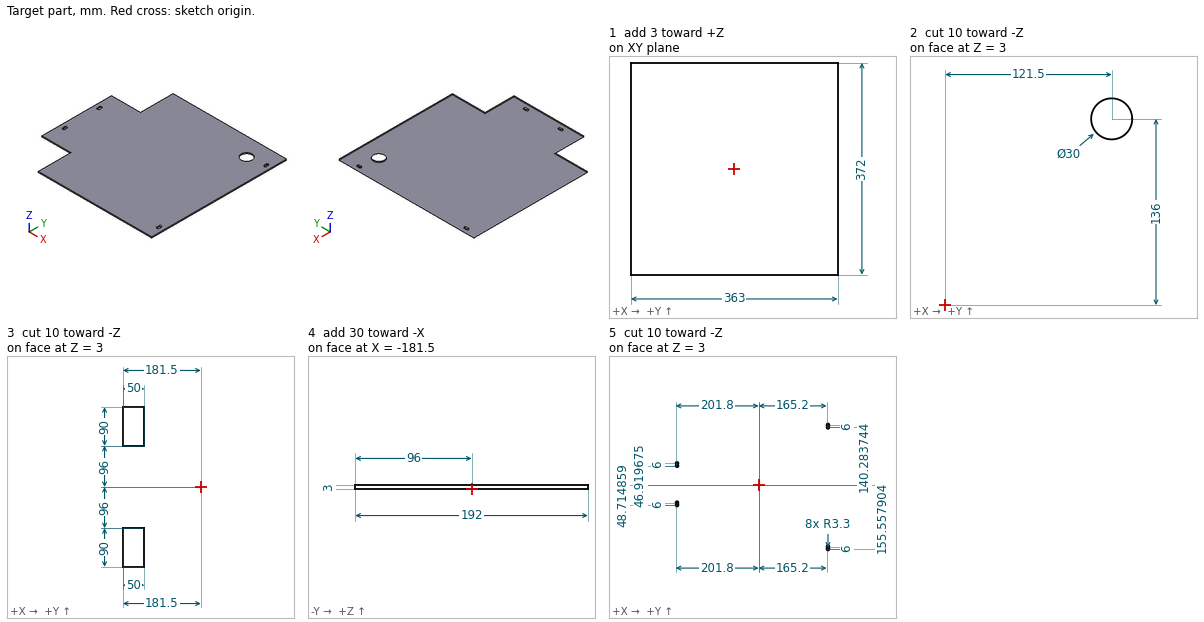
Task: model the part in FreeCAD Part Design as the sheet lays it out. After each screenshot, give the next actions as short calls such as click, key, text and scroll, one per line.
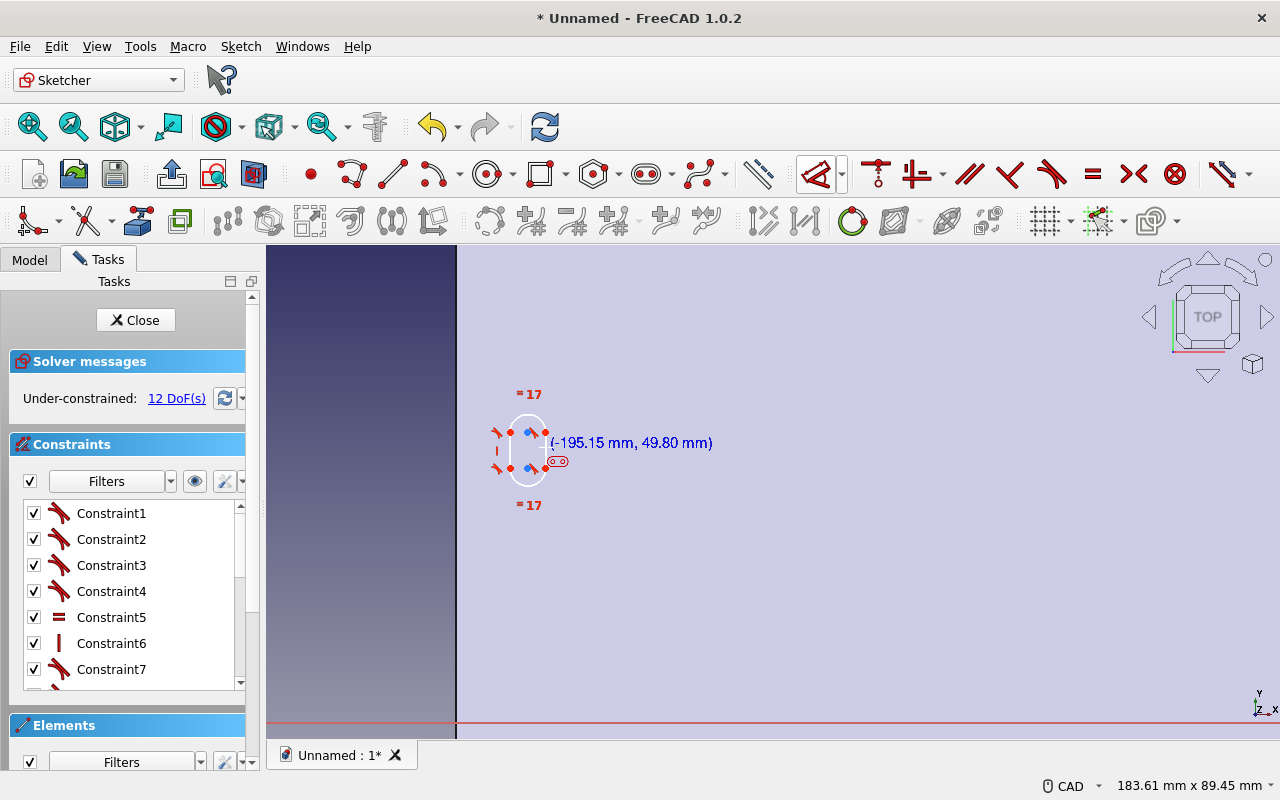
scroll(539, 441, down, 9)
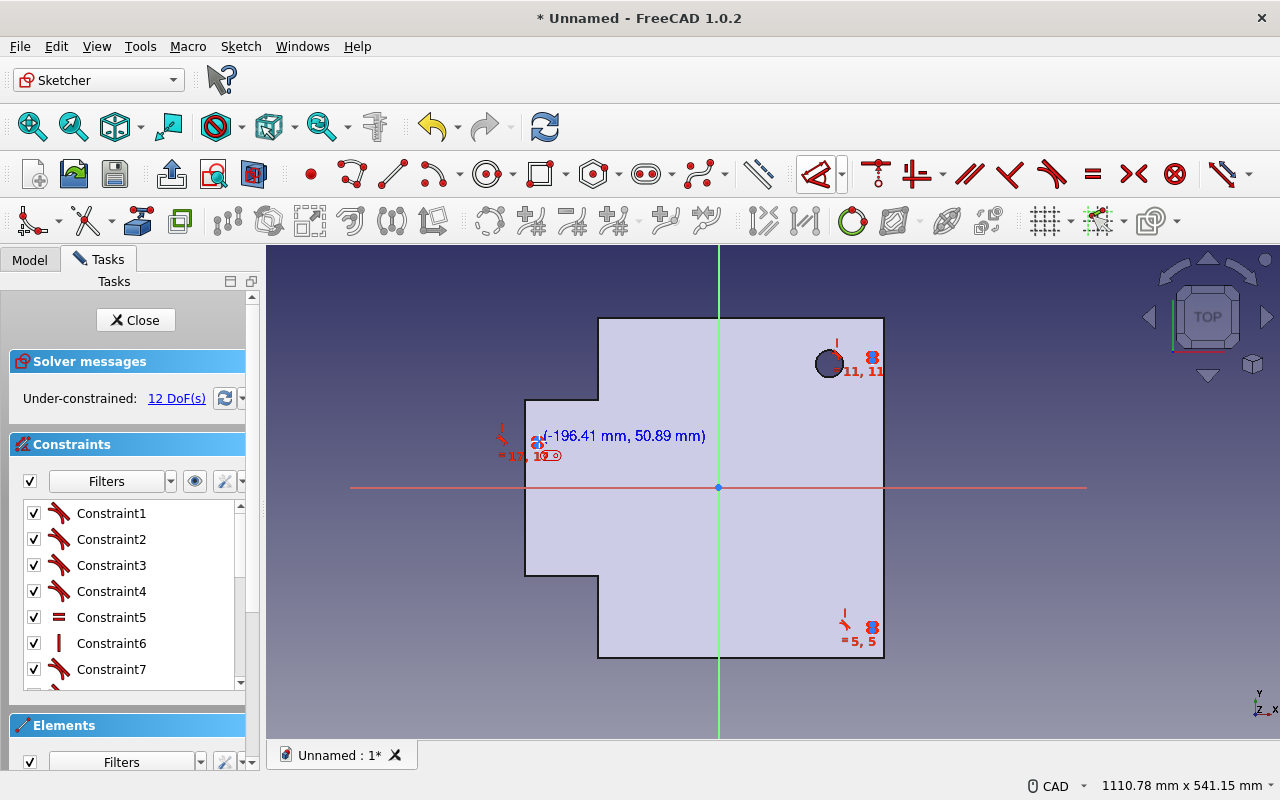
scroll(537, 532, up, 11)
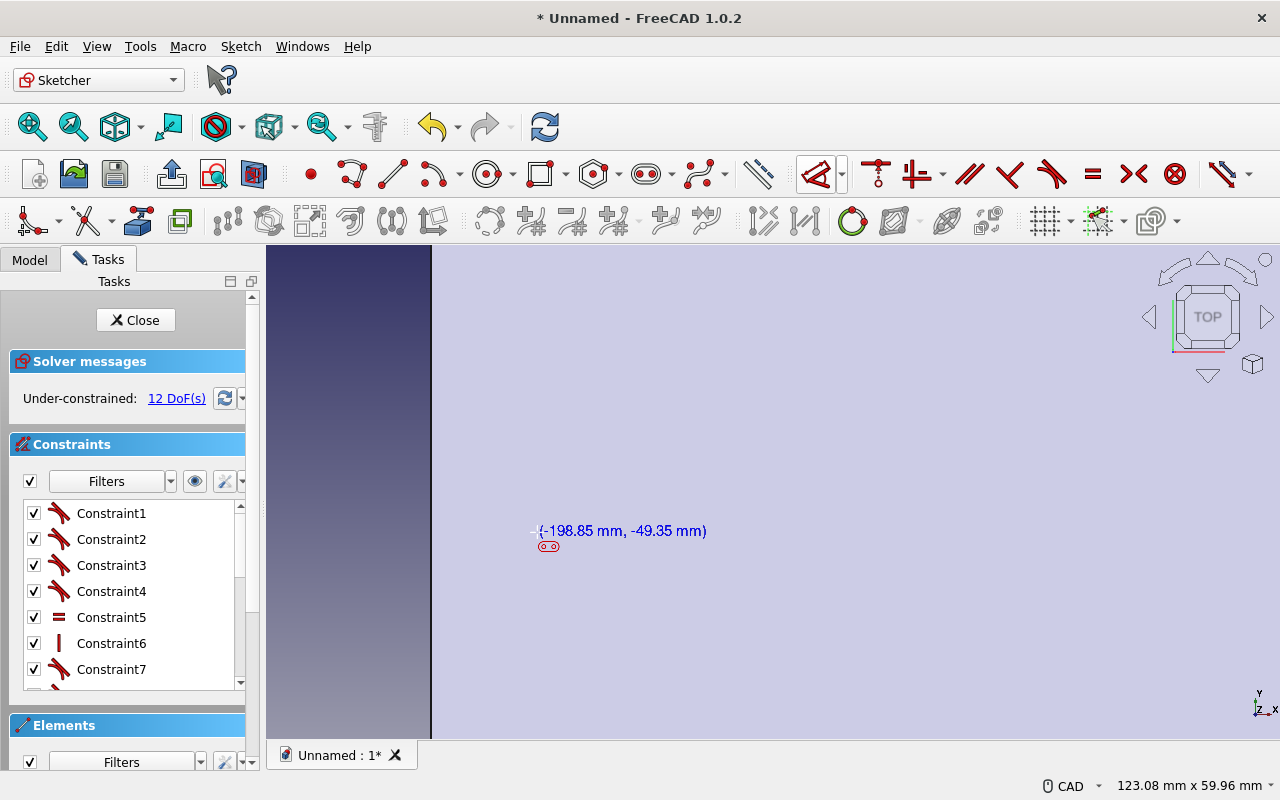
scroll(537, 532, down, 11)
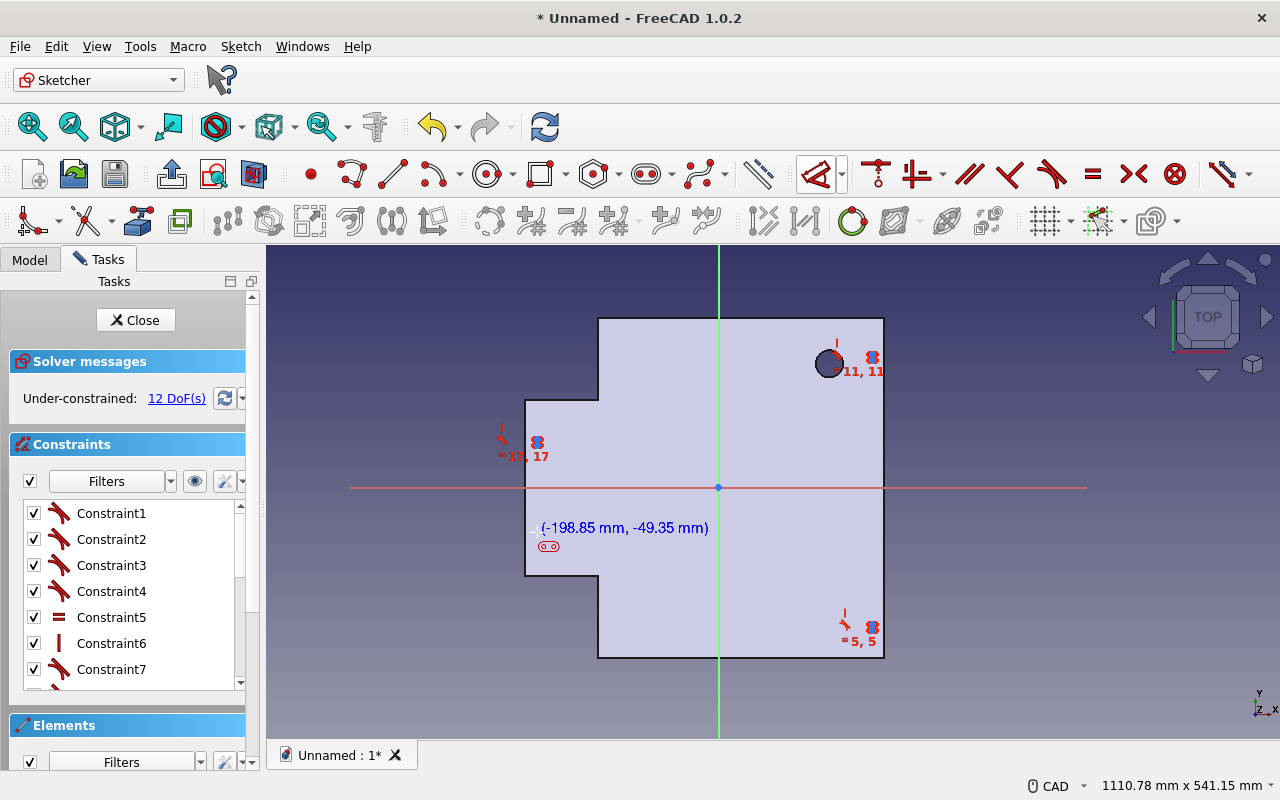
click(537, 532)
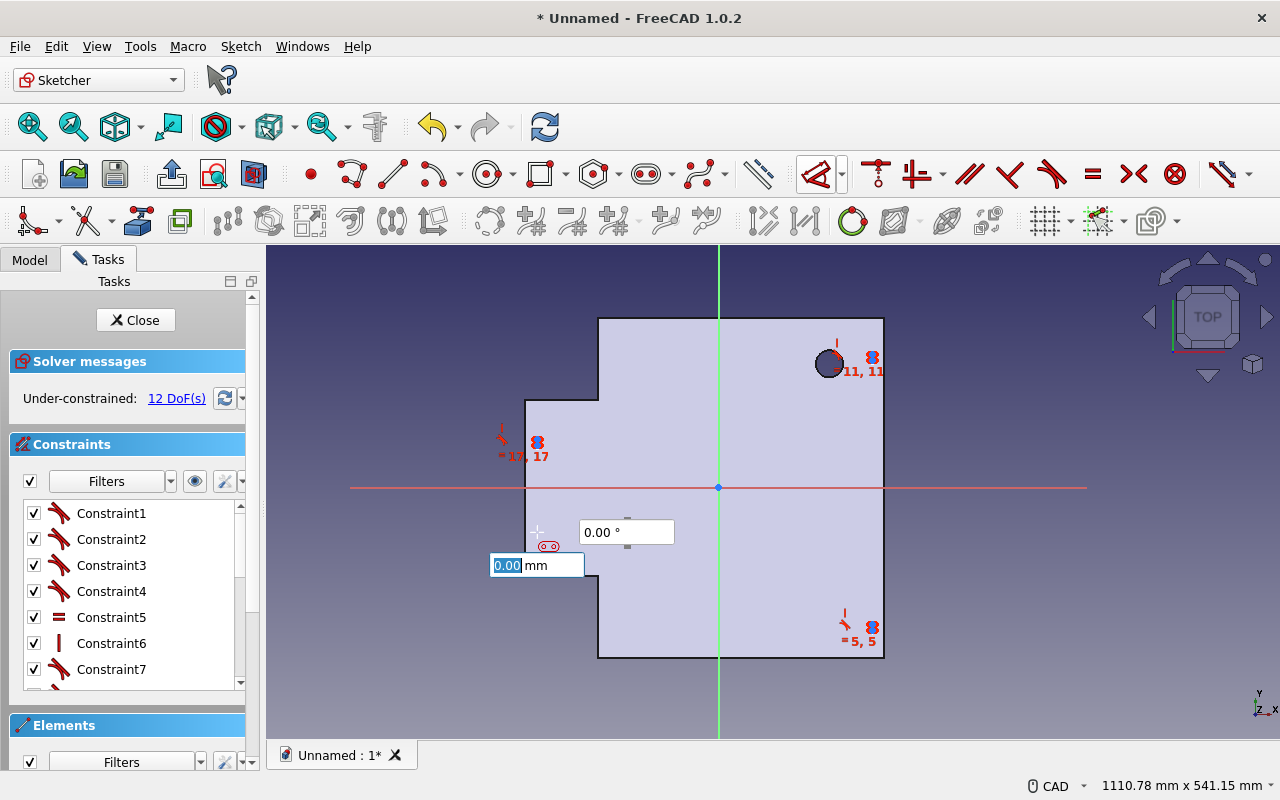
scroll(537, 527, up, 6)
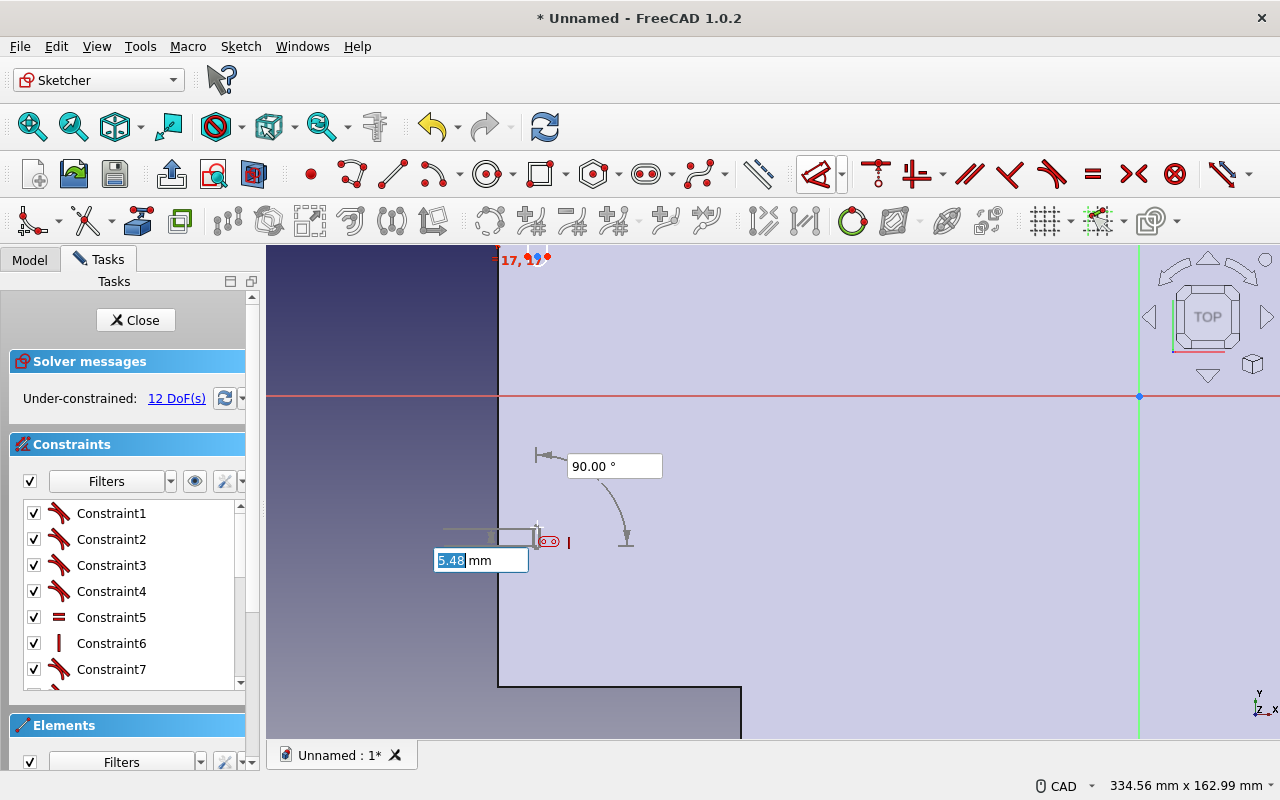
click(536, 525)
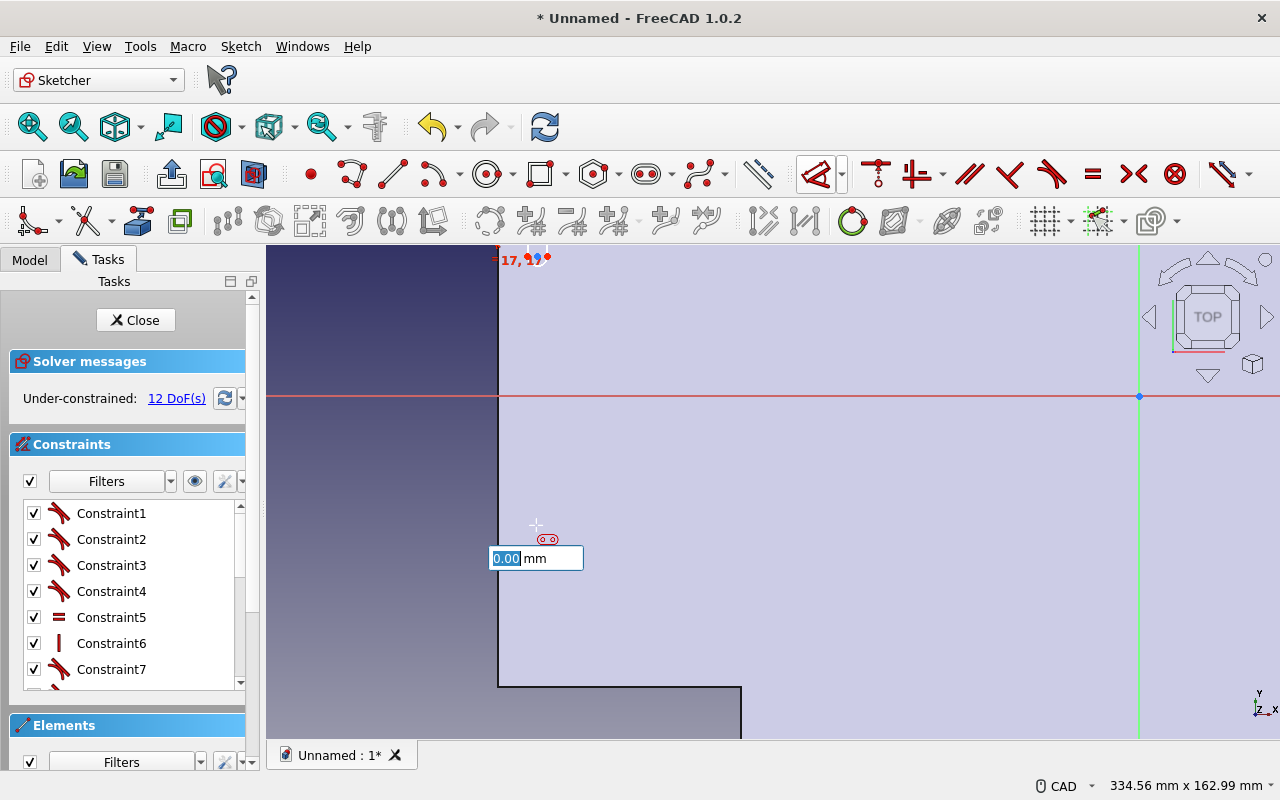
scroll(527, 535, up, 3)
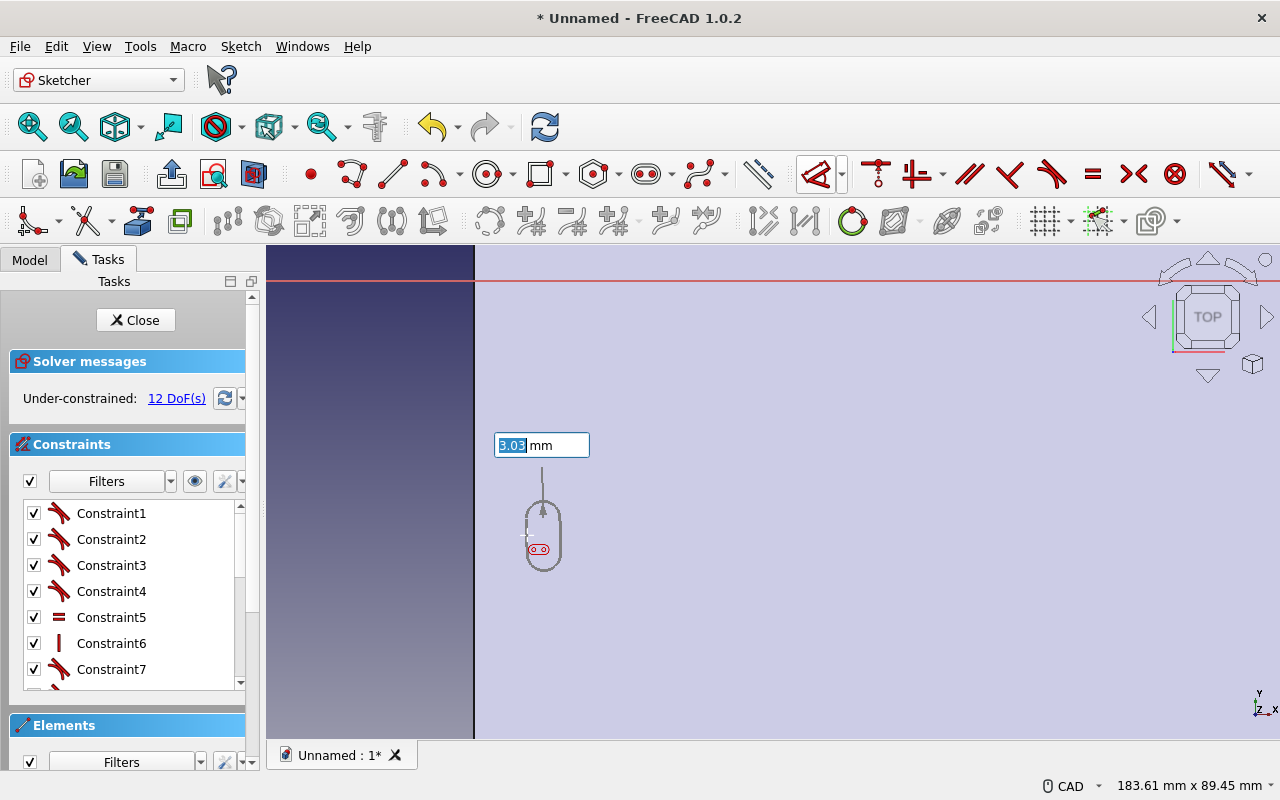
click(528, 534)
key(Escape)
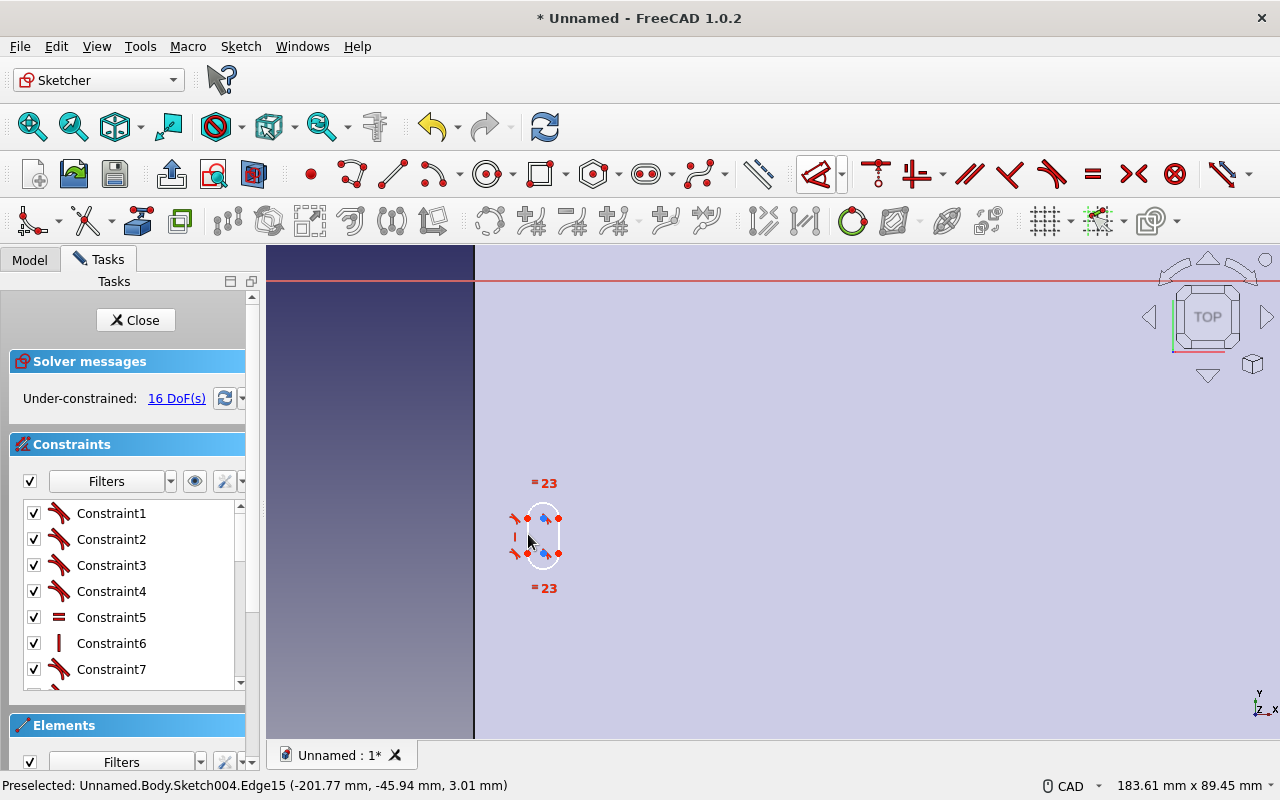
scroll(535, 529, down, 9)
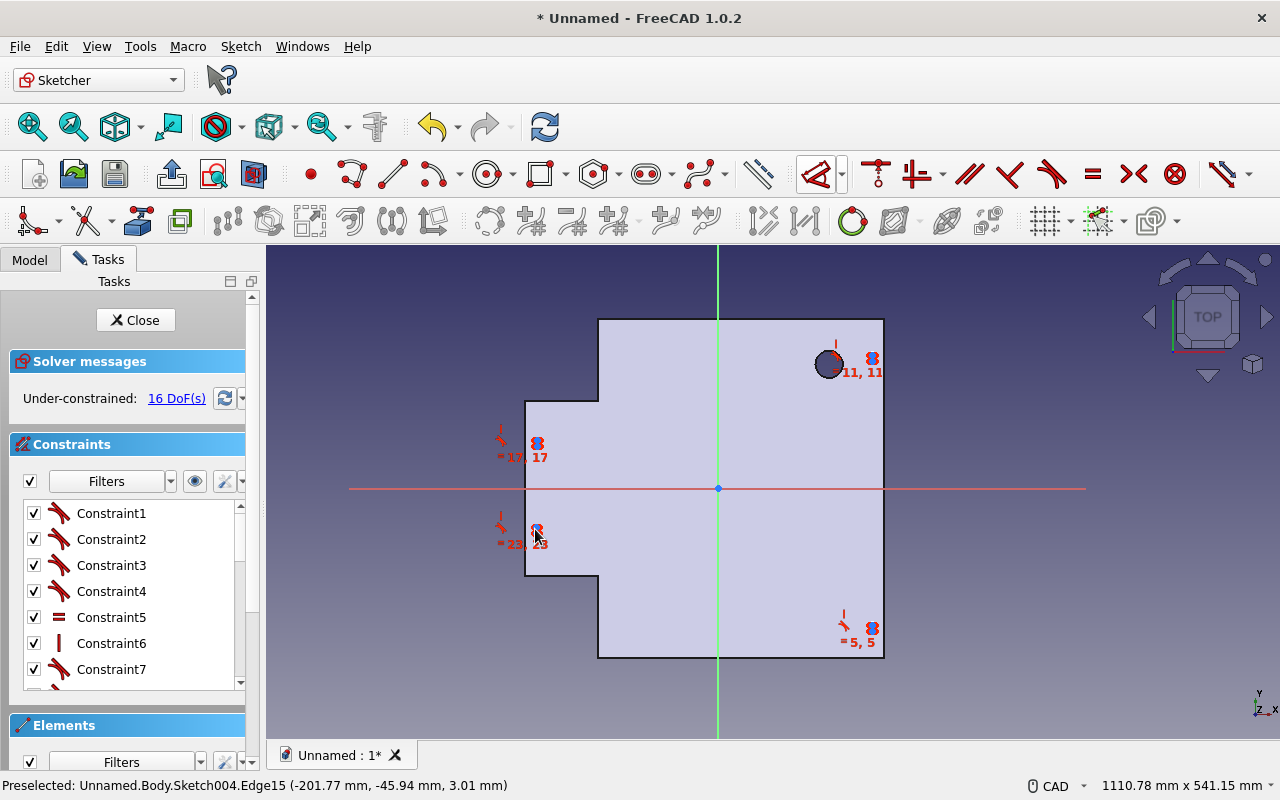
scroll(870, 634, up, 8)